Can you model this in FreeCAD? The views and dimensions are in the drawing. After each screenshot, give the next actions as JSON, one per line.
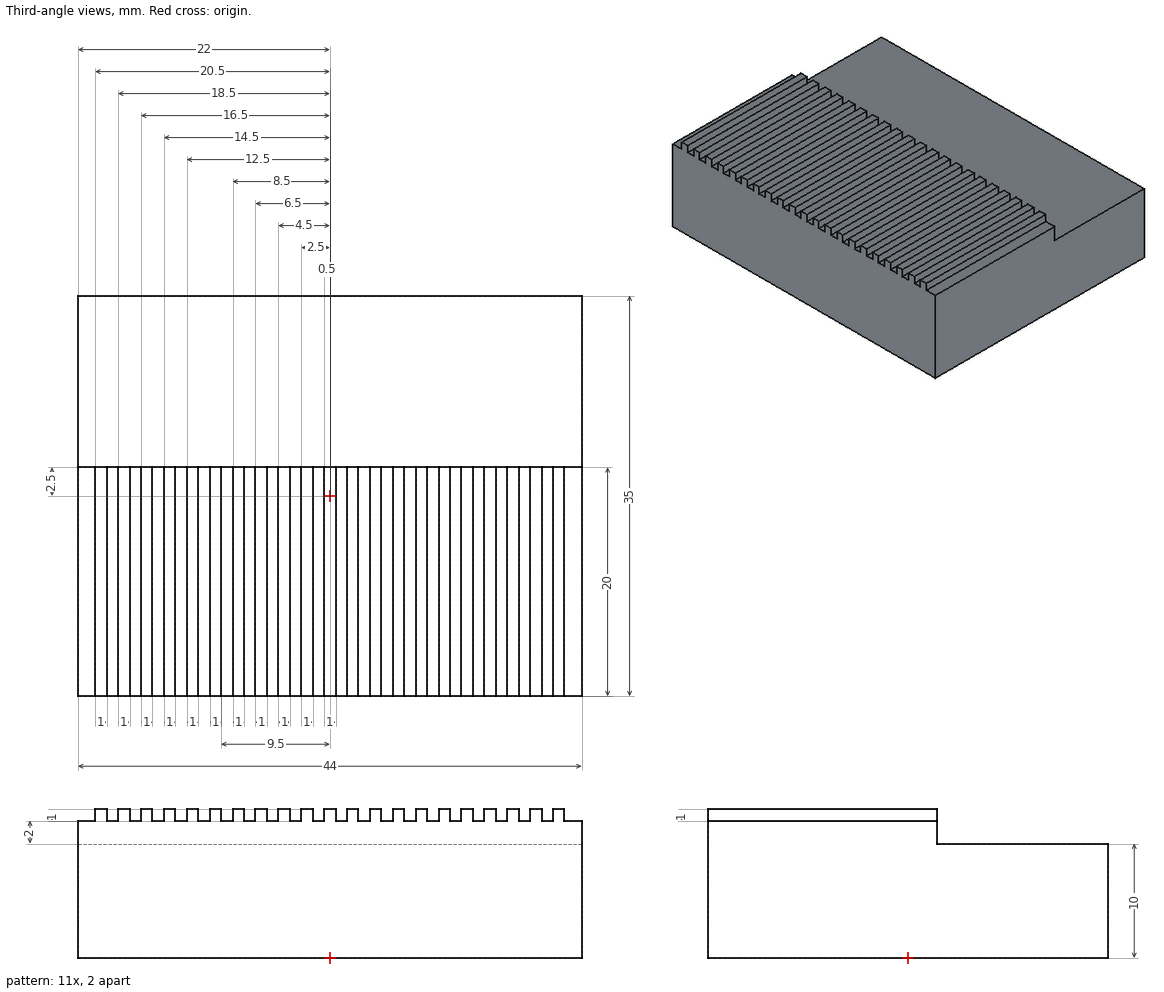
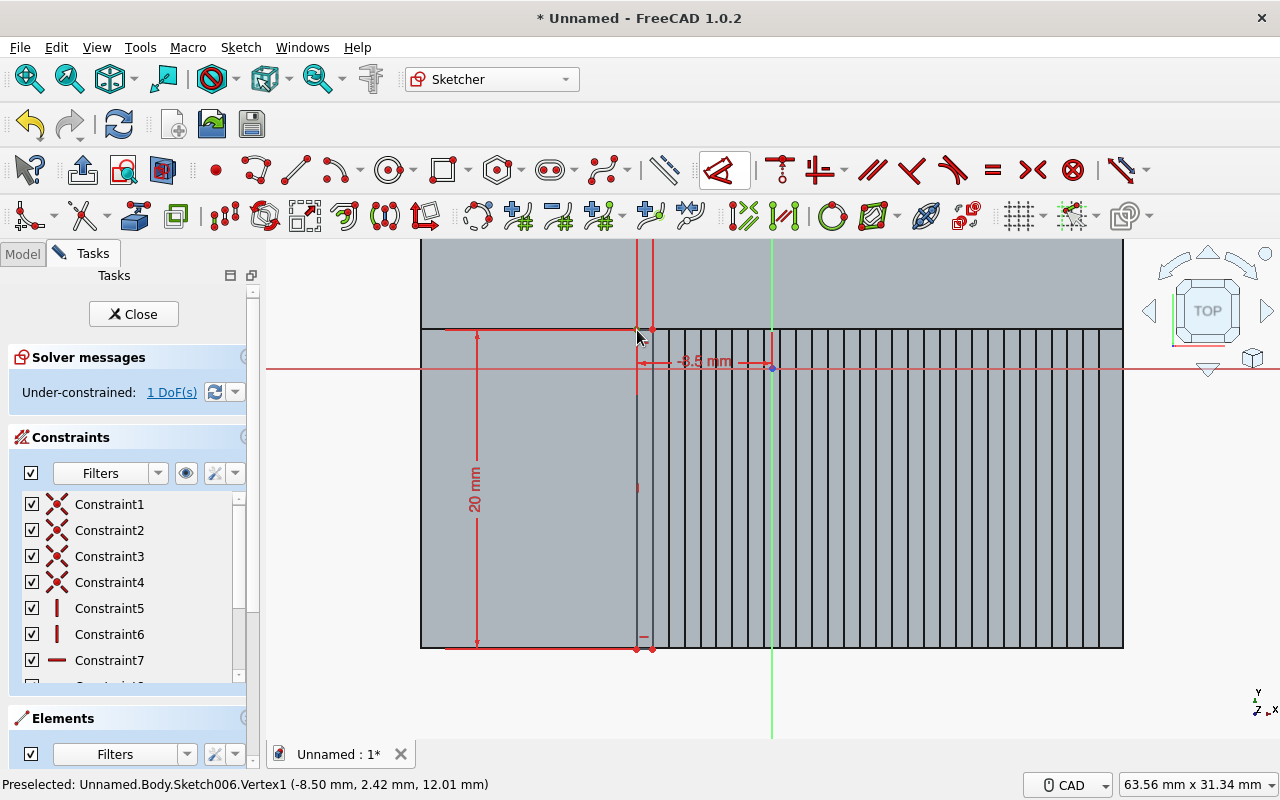
{"action": "left_click", "coordinate": [744, 170]}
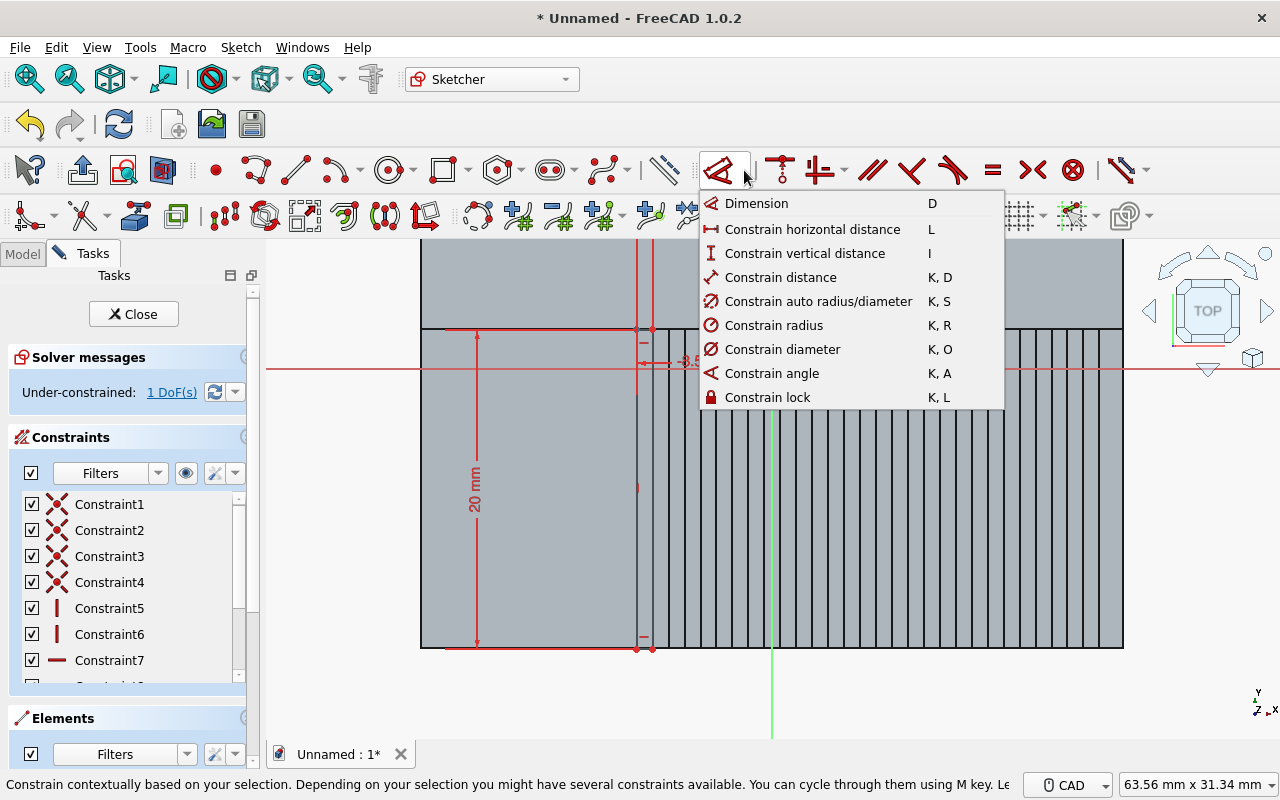
{"action": "left_click", "coordinate": [852, 253]}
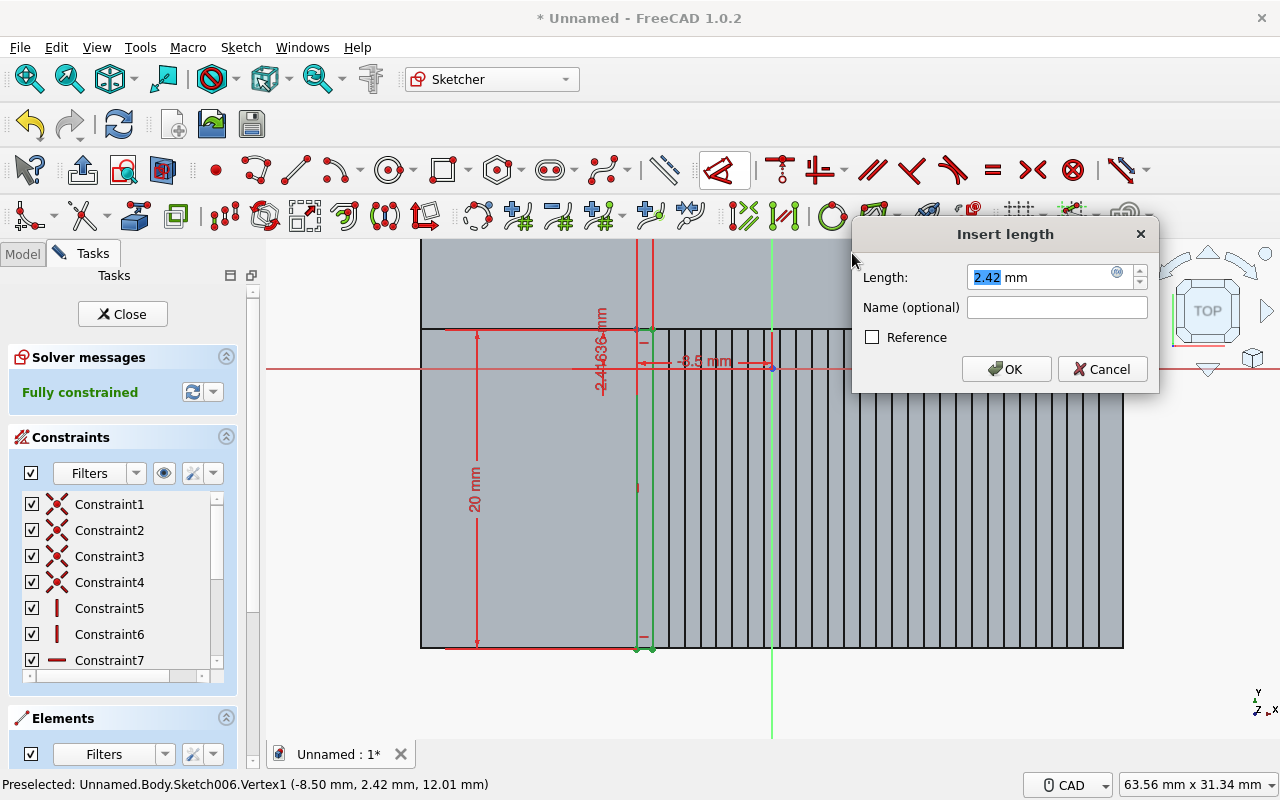
{"action": "type", "text": "2.5"}
{"action": "key", "text": "Return"}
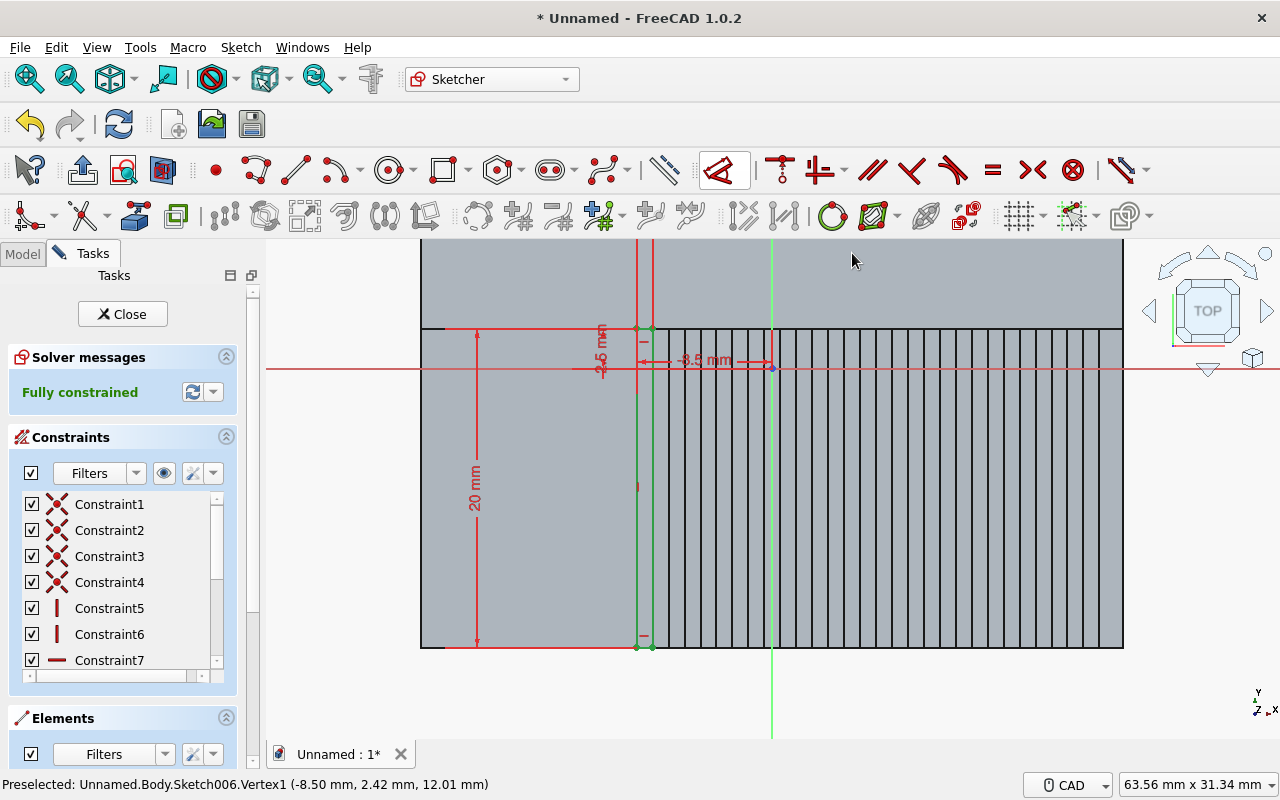
{"action": "left_click", "coordinate": [123, 314]}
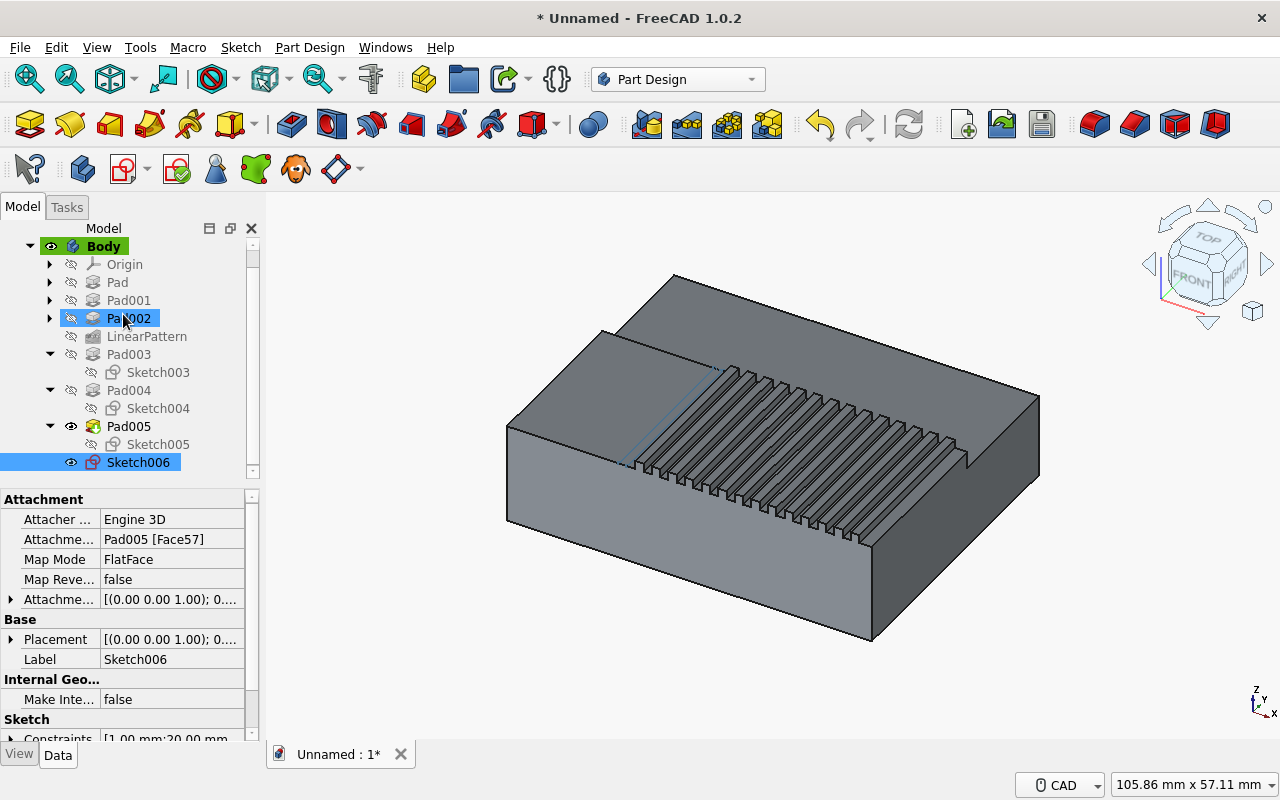
{"action": "left_click", "coordinate": [30, 124]}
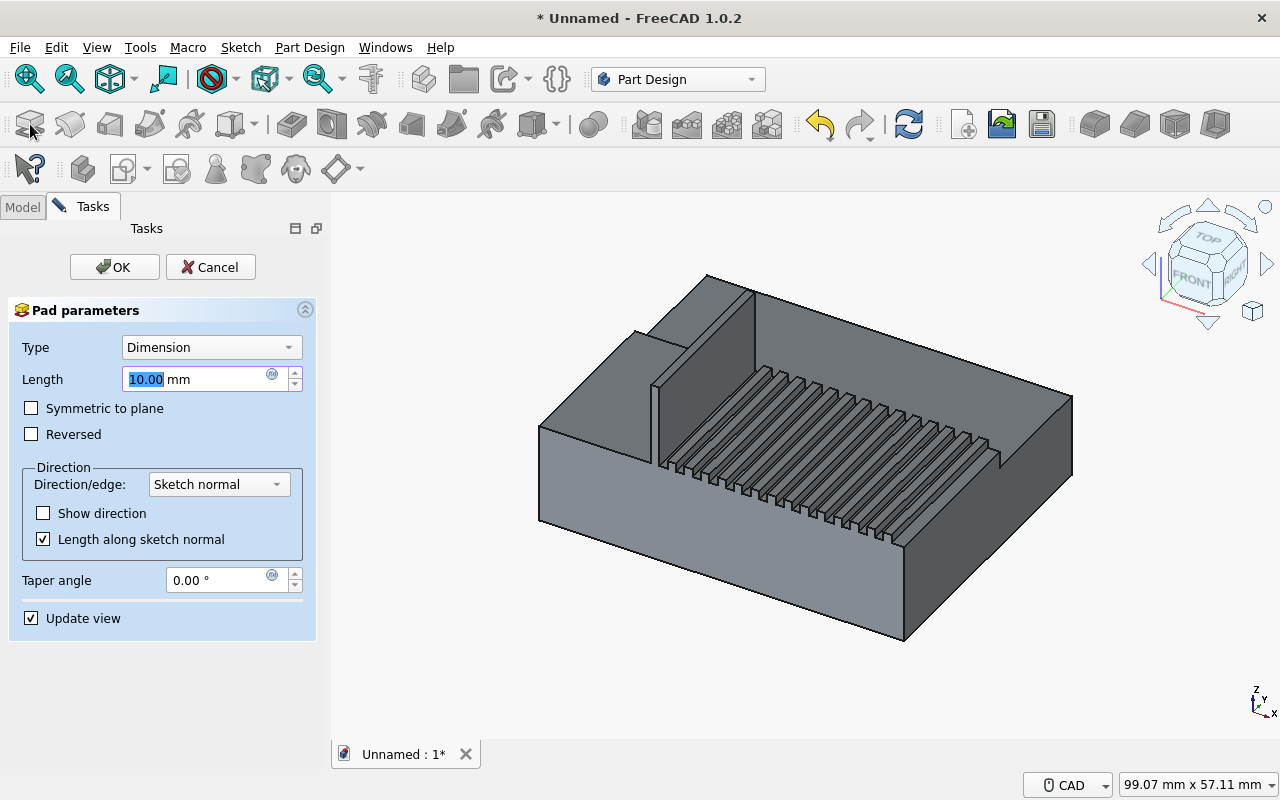
{"action": "type", "text": "1"}
{"action": "key", "text": "Tab"}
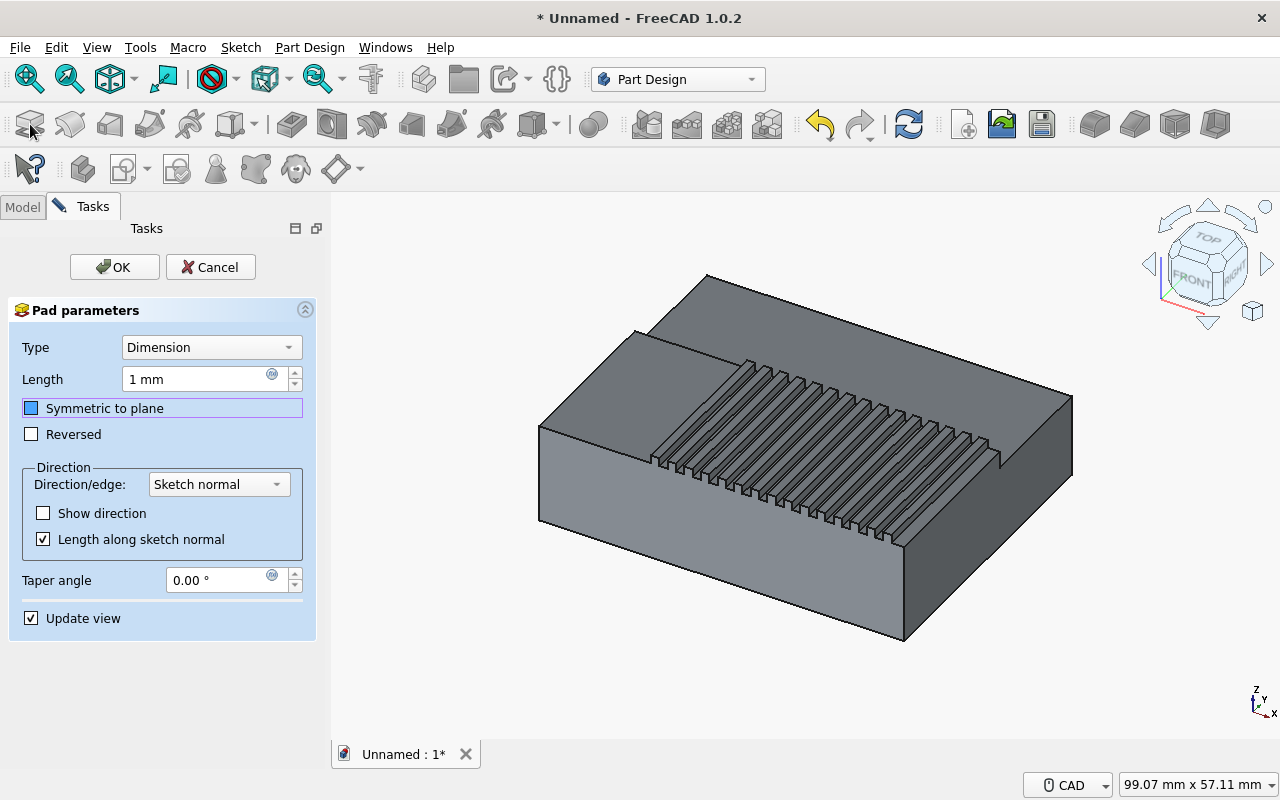
{"action": "left_click", "coordinate": [115, 267]}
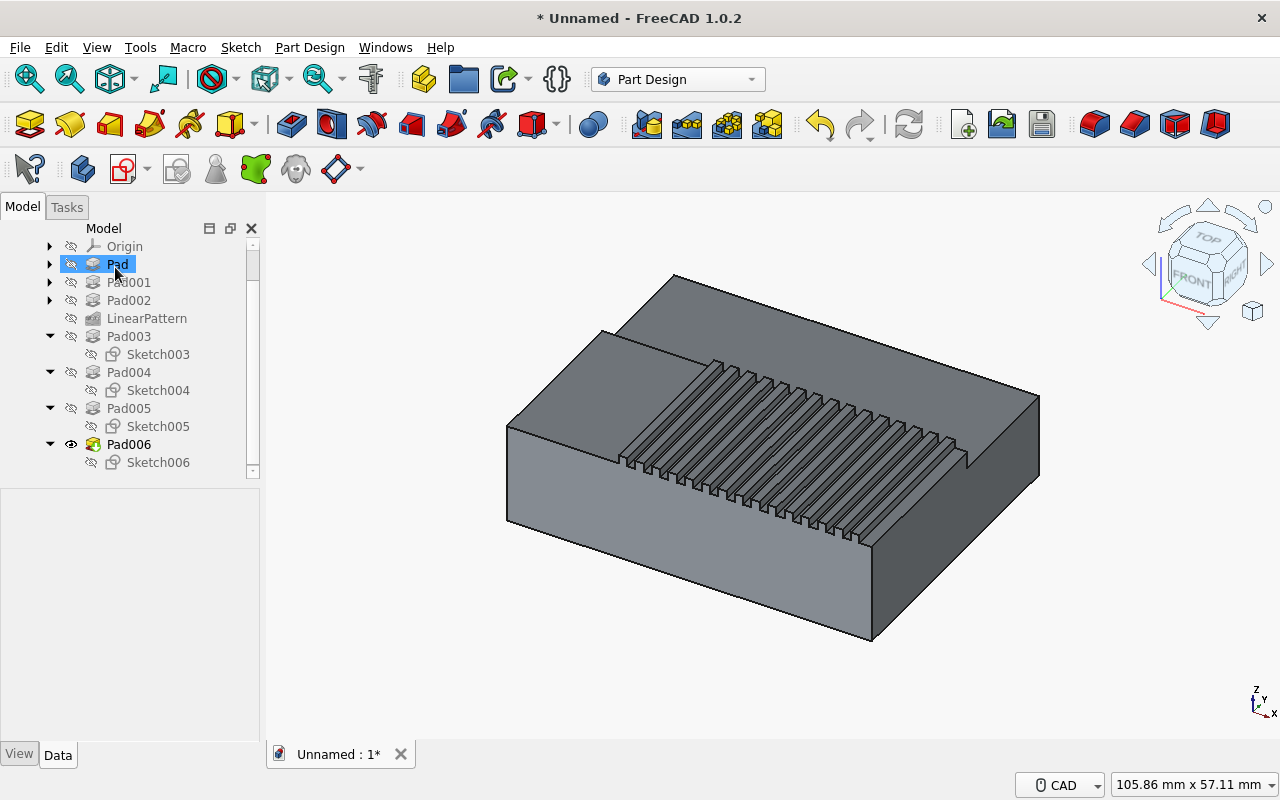
{"action": "left_click", "coordinate": [624, 383]}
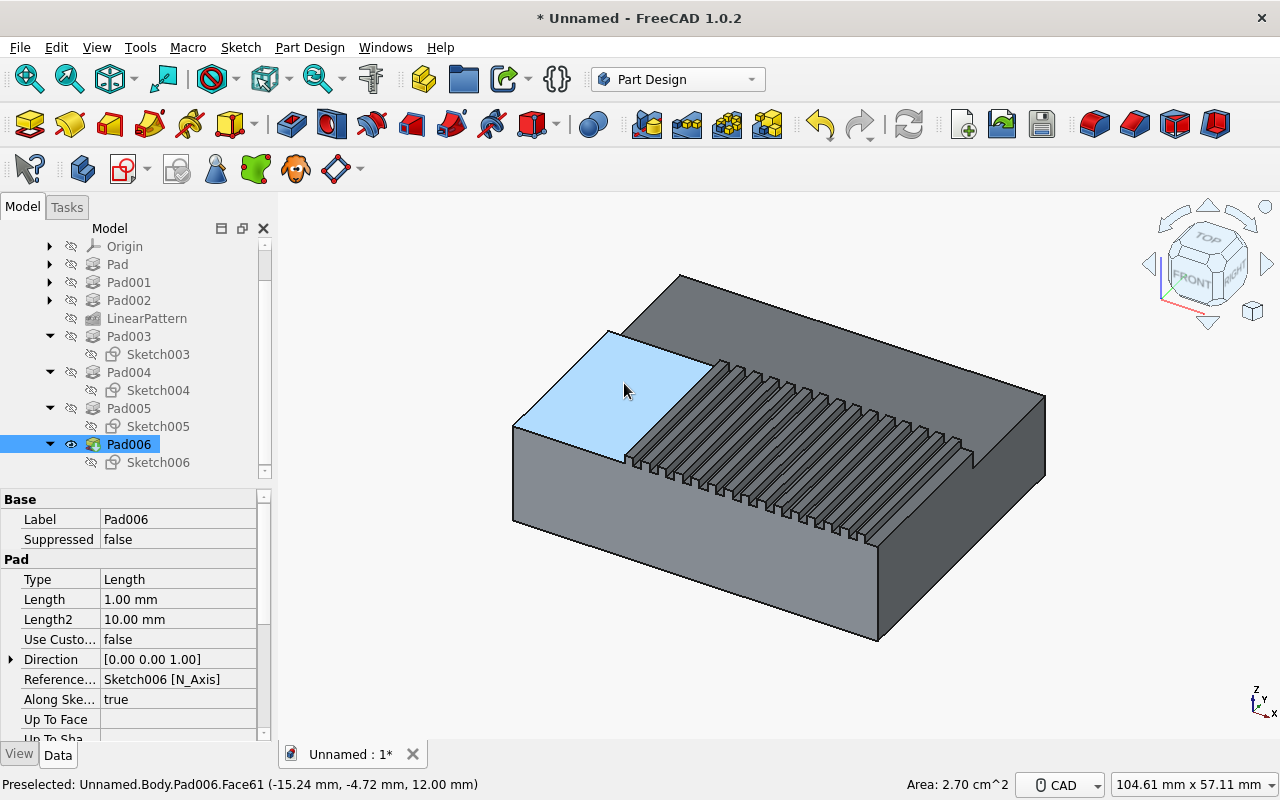
{"action": "left_click", "coordinate": [124, 170]}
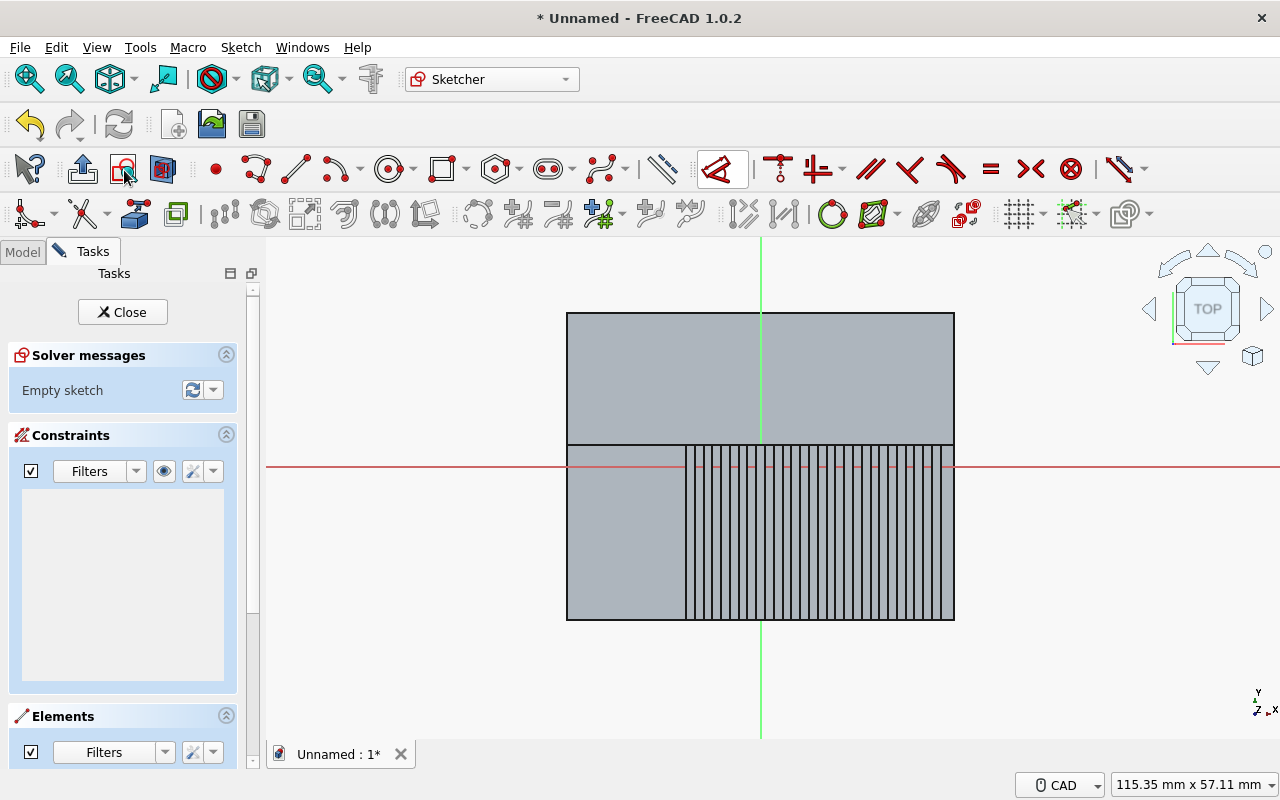
{"action": "scroll", "coordinate": [727, 587], "scroll_direction": "up", "scroll_amount": 3}